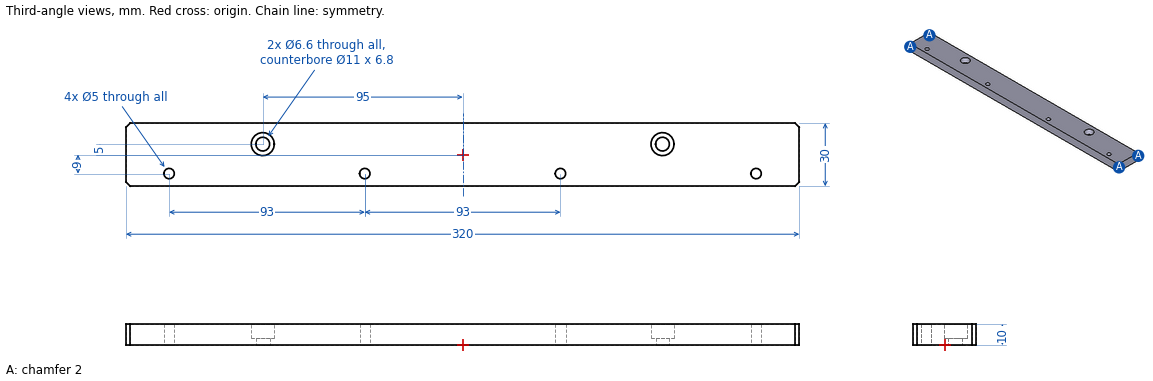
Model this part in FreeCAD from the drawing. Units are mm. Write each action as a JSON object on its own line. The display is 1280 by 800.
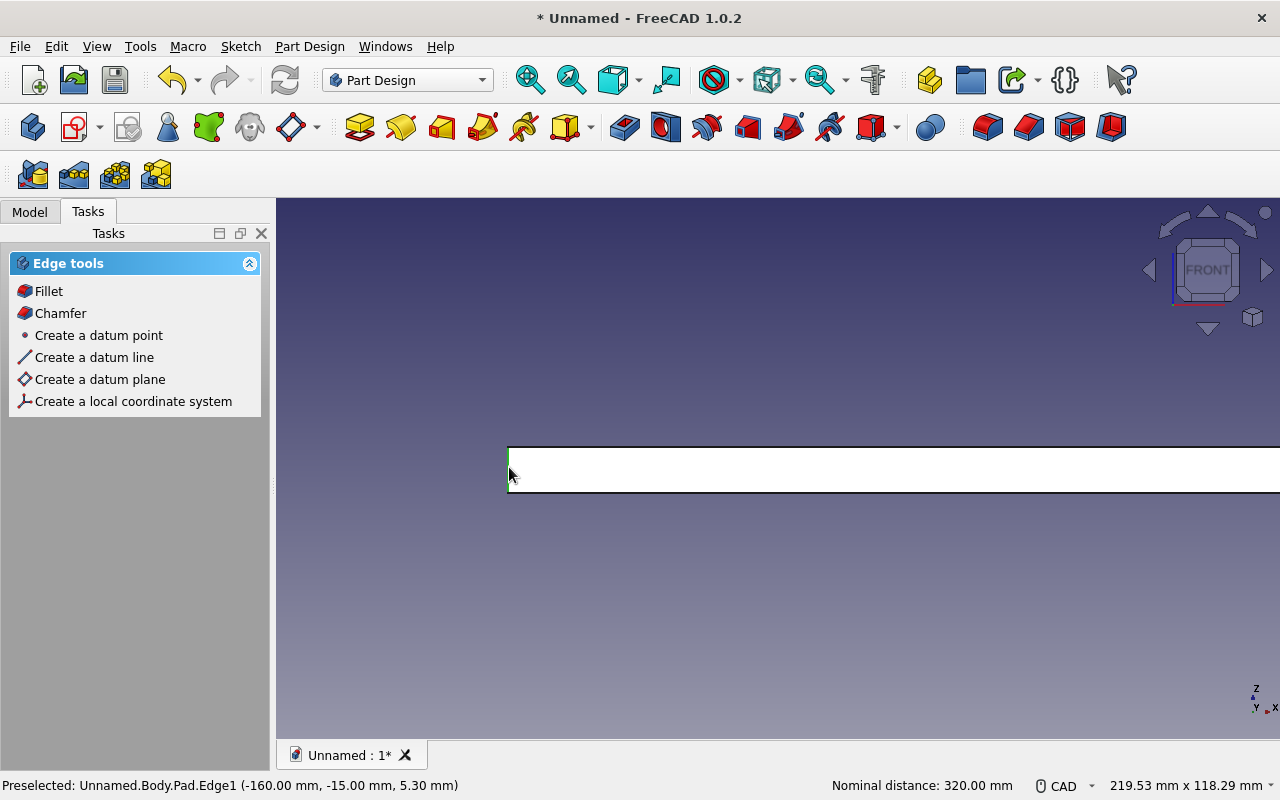
{"action": "left_click", "coordinate": [531, 80]}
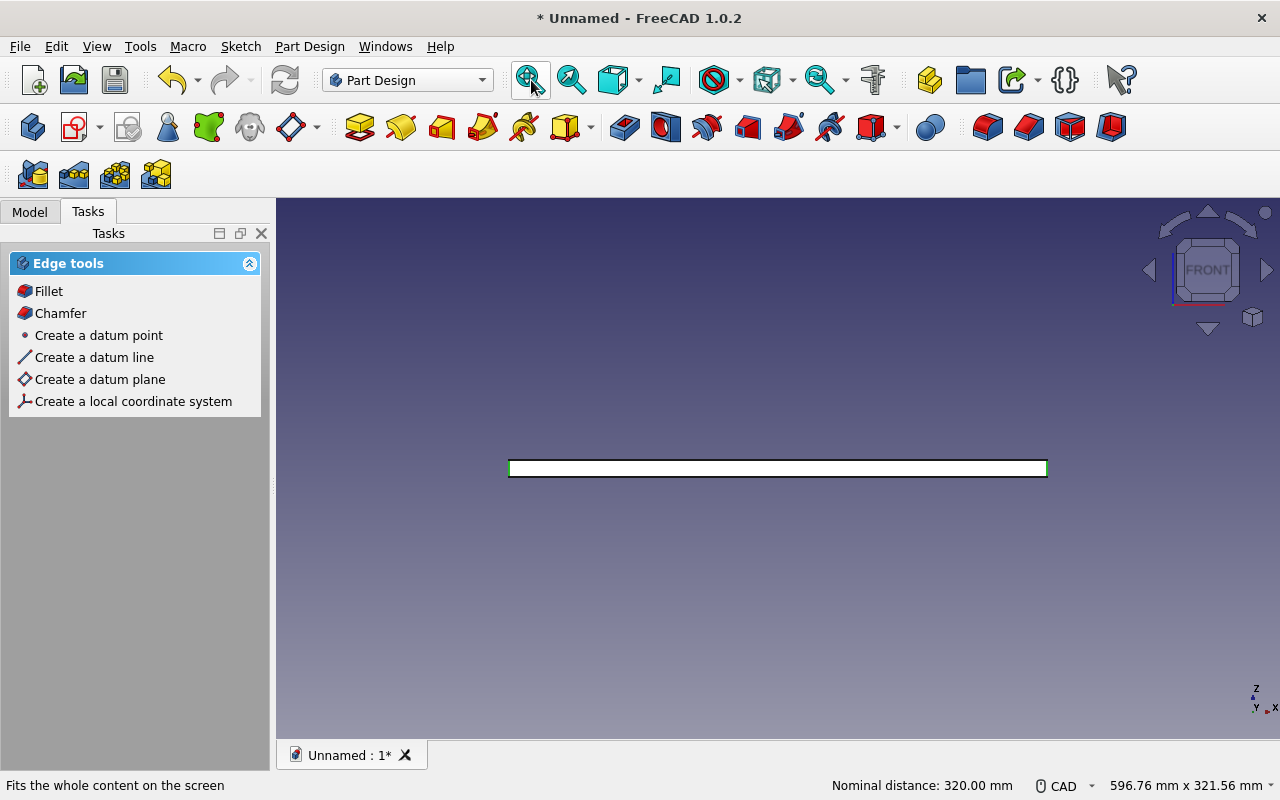
{"action": "key", "text": "3"}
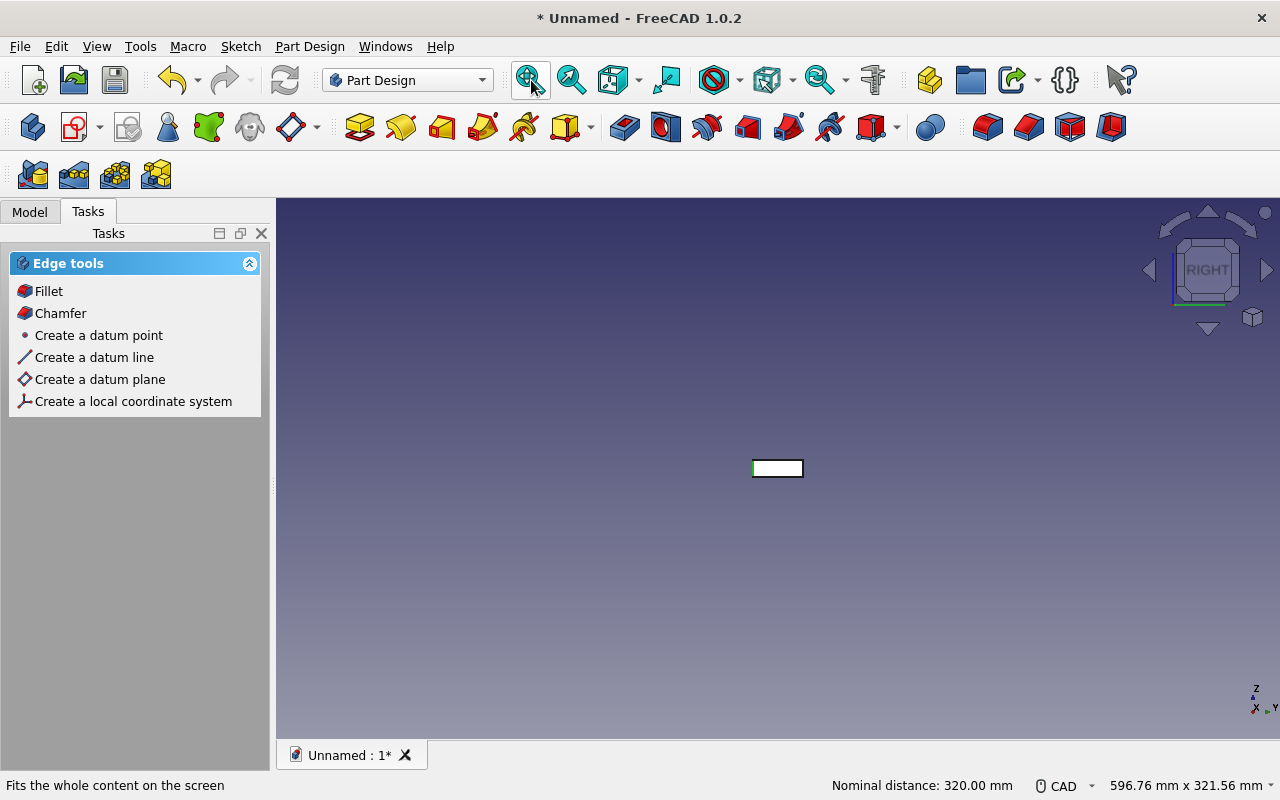
{"action": "left_click", "coordinate": [531, 80]}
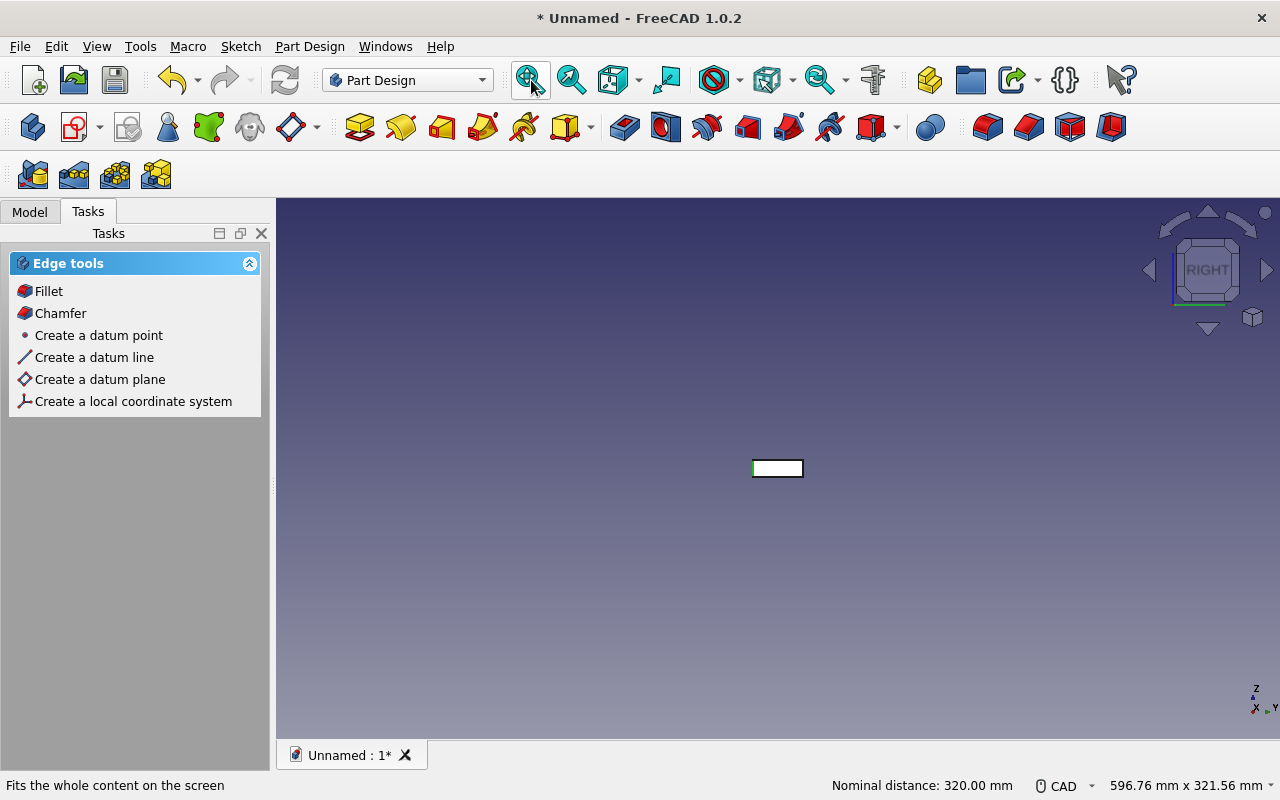
{"action": "left_click", "coordinate": [803, 467], "text": "ctrl"}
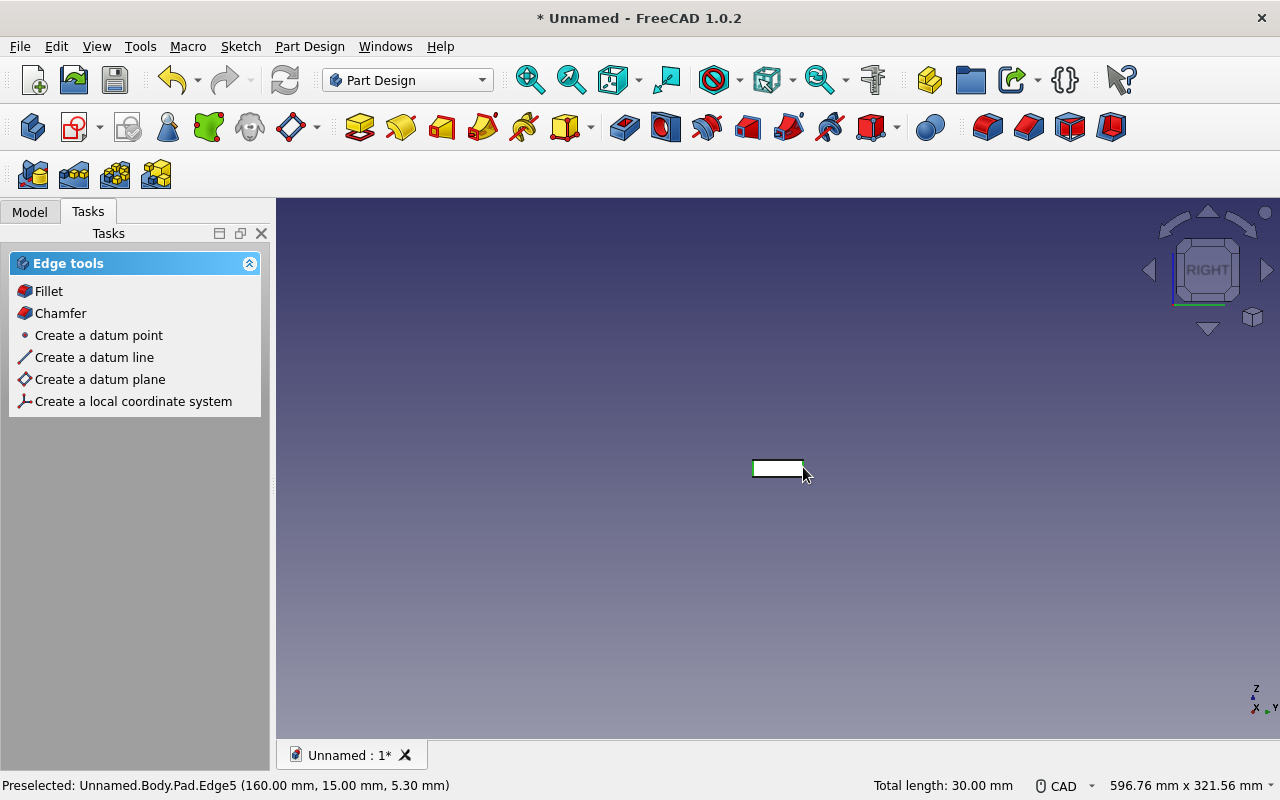
{"action": "scroll", "coordinate": [803, 467], "scroll_direction": "up", "scroll_amount": 5}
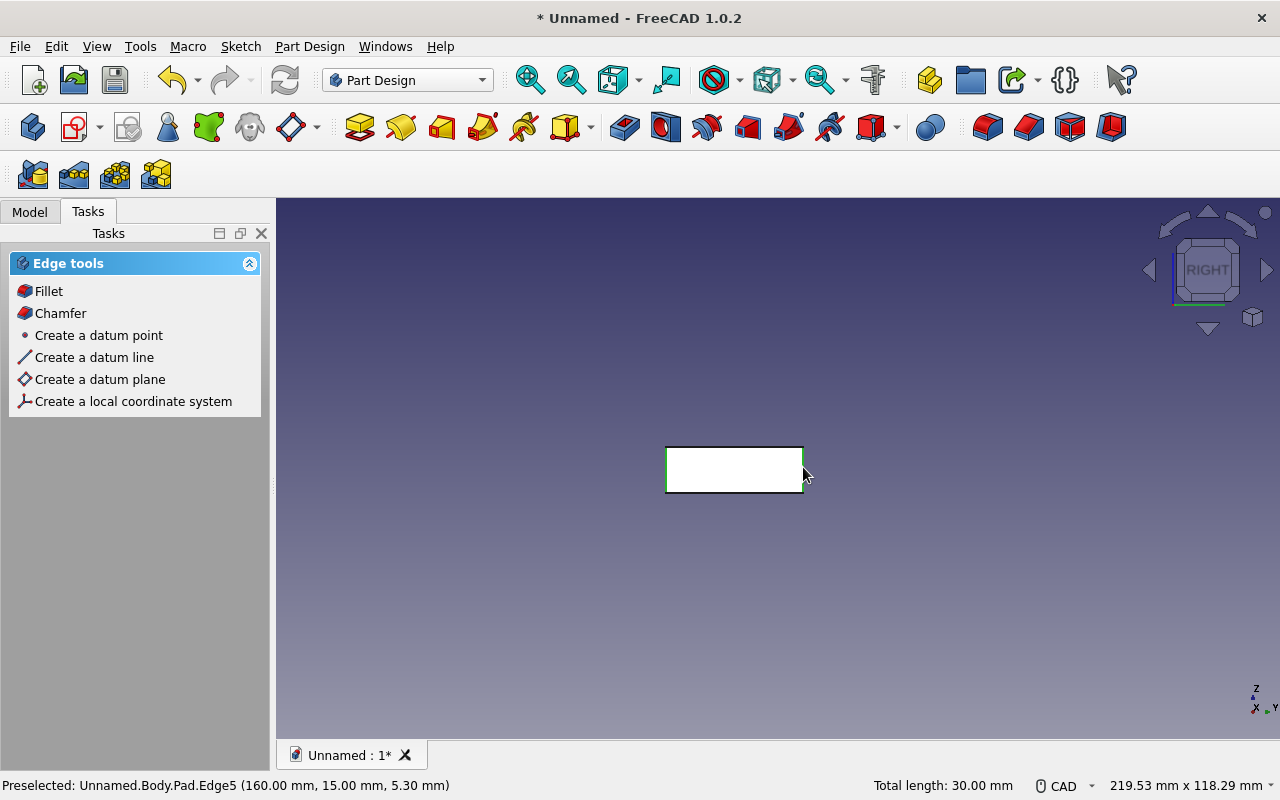
{"action": "left_click", "coordinate": [531, 80]}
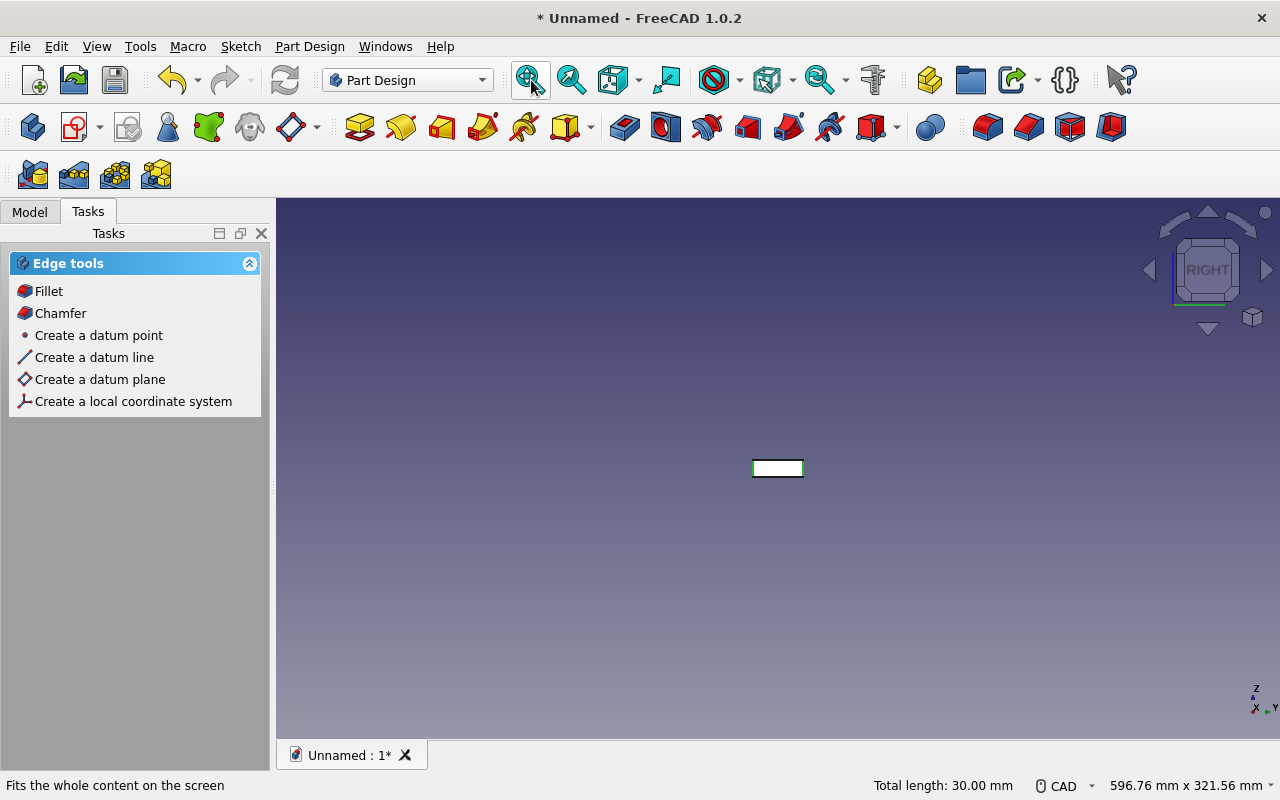
{"action": "key", "text": "5"}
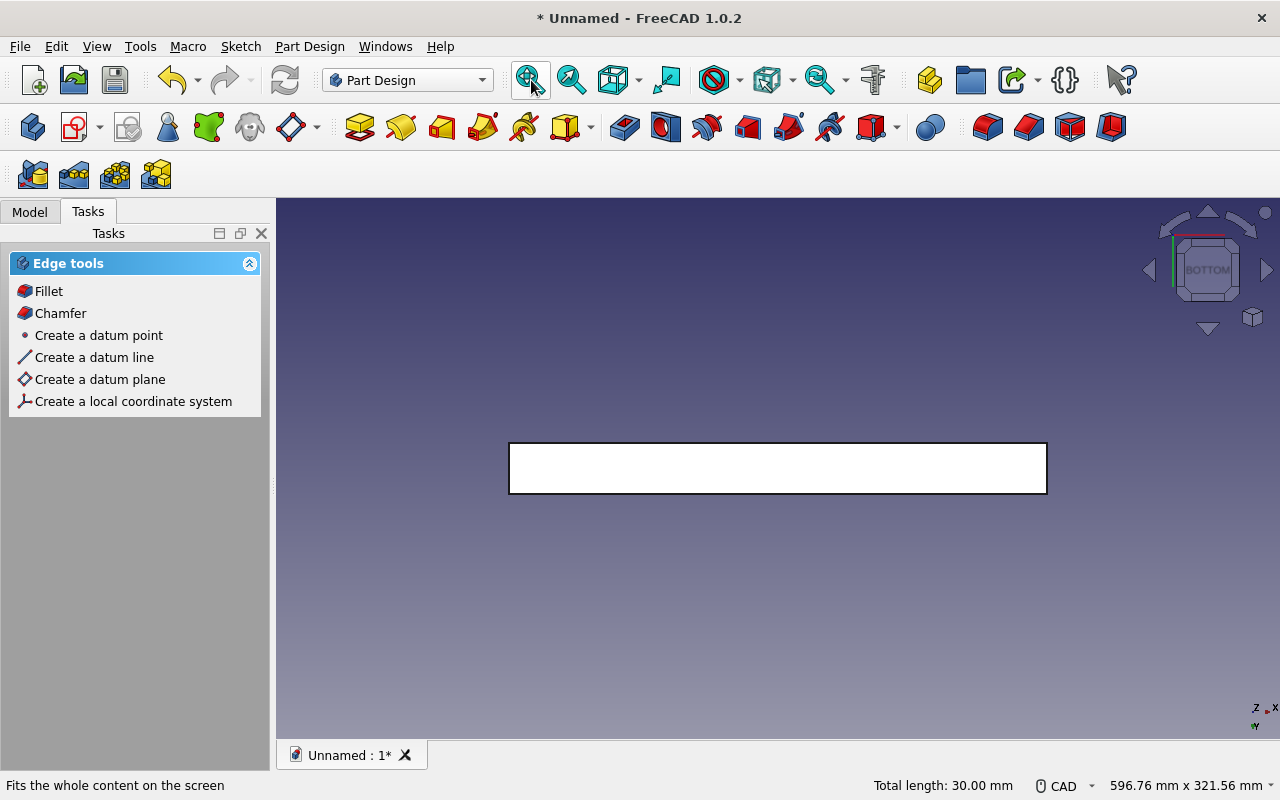
{"action": "scroll", "coordinate": [509, 493], "scroll_direction": "up", "scroll_amount": 5}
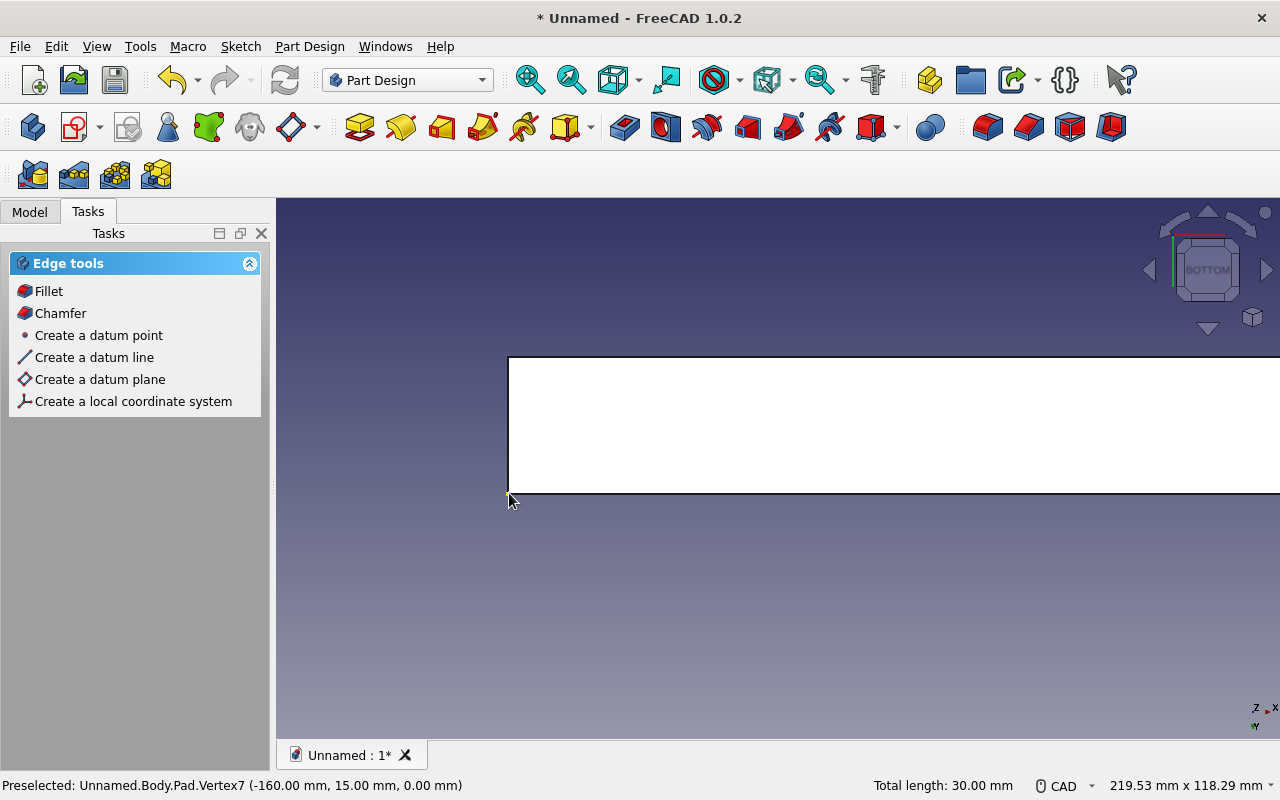
{"action": "left_click", "coordinate": [531, 80]}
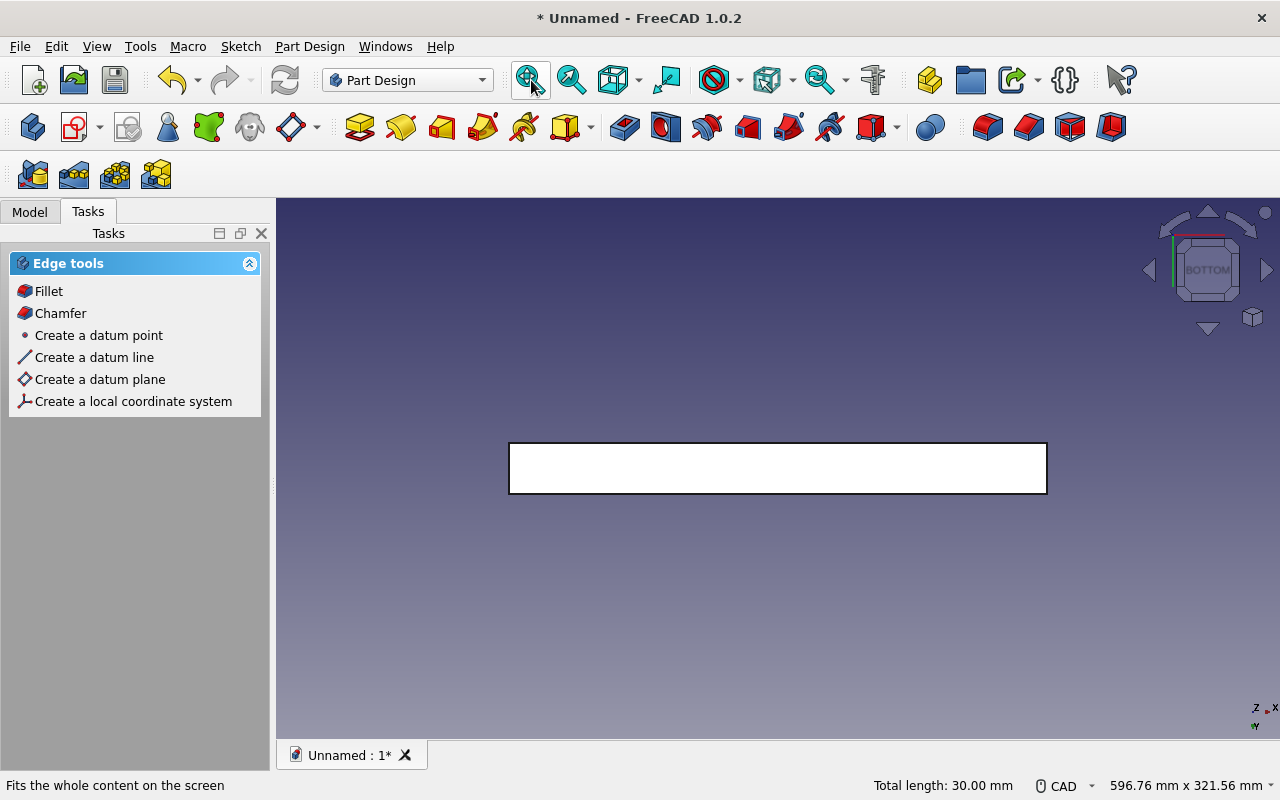
{"action": "key", "text": "4"}